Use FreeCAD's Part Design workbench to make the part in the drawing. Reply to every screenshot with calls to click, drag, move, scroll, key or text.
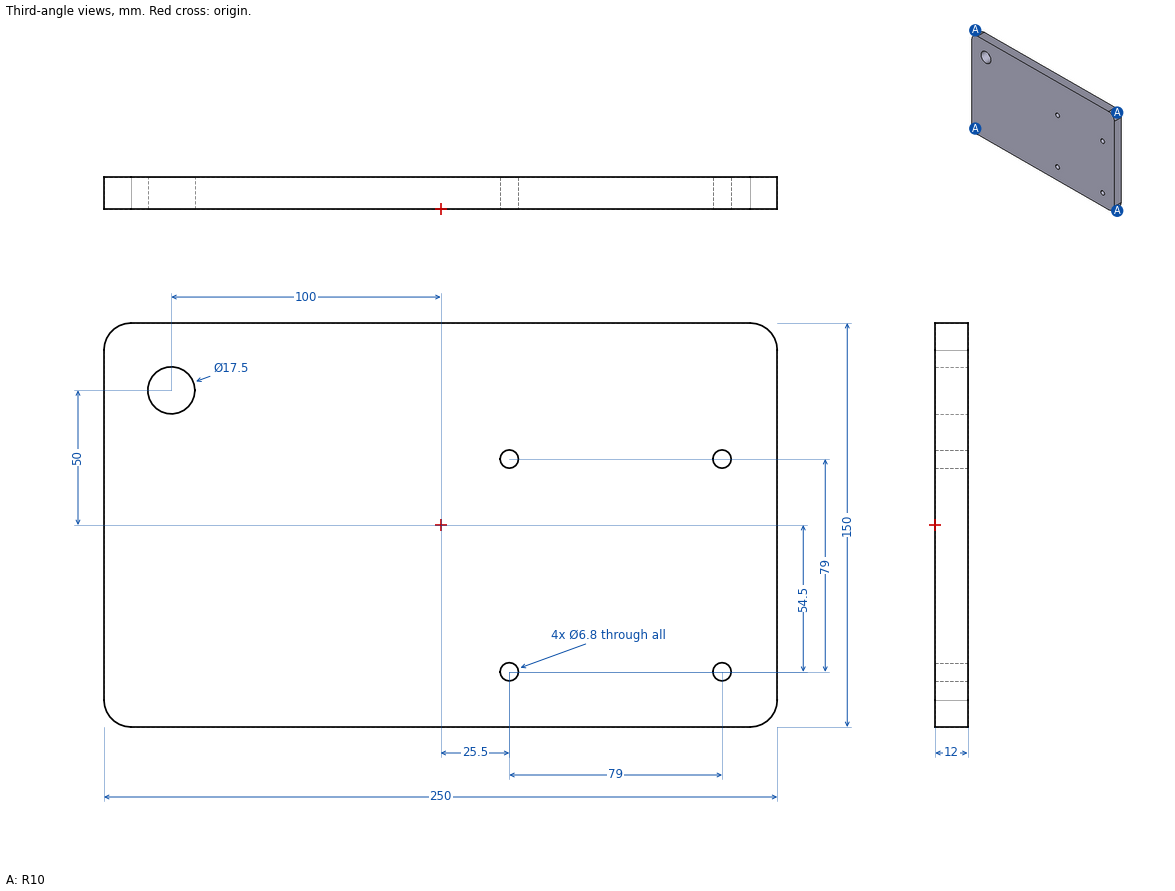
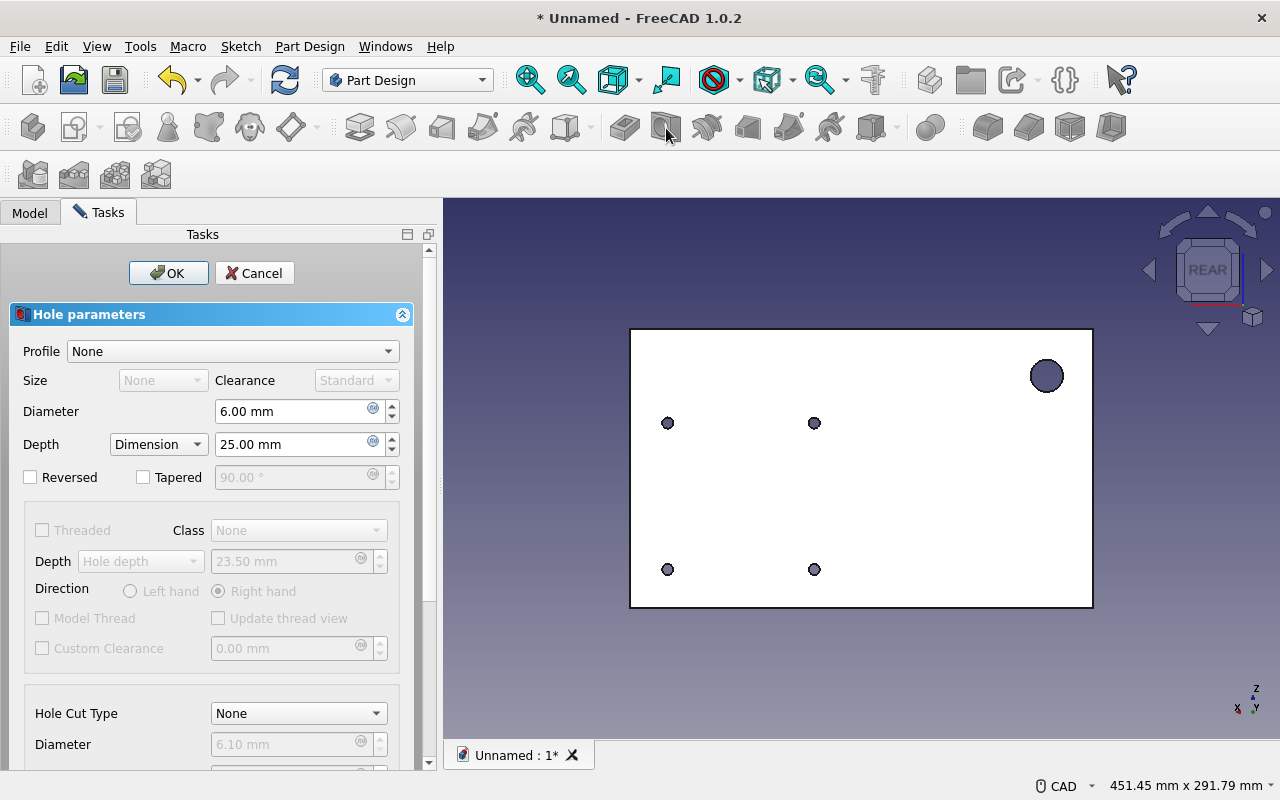
triple_click(300, 412)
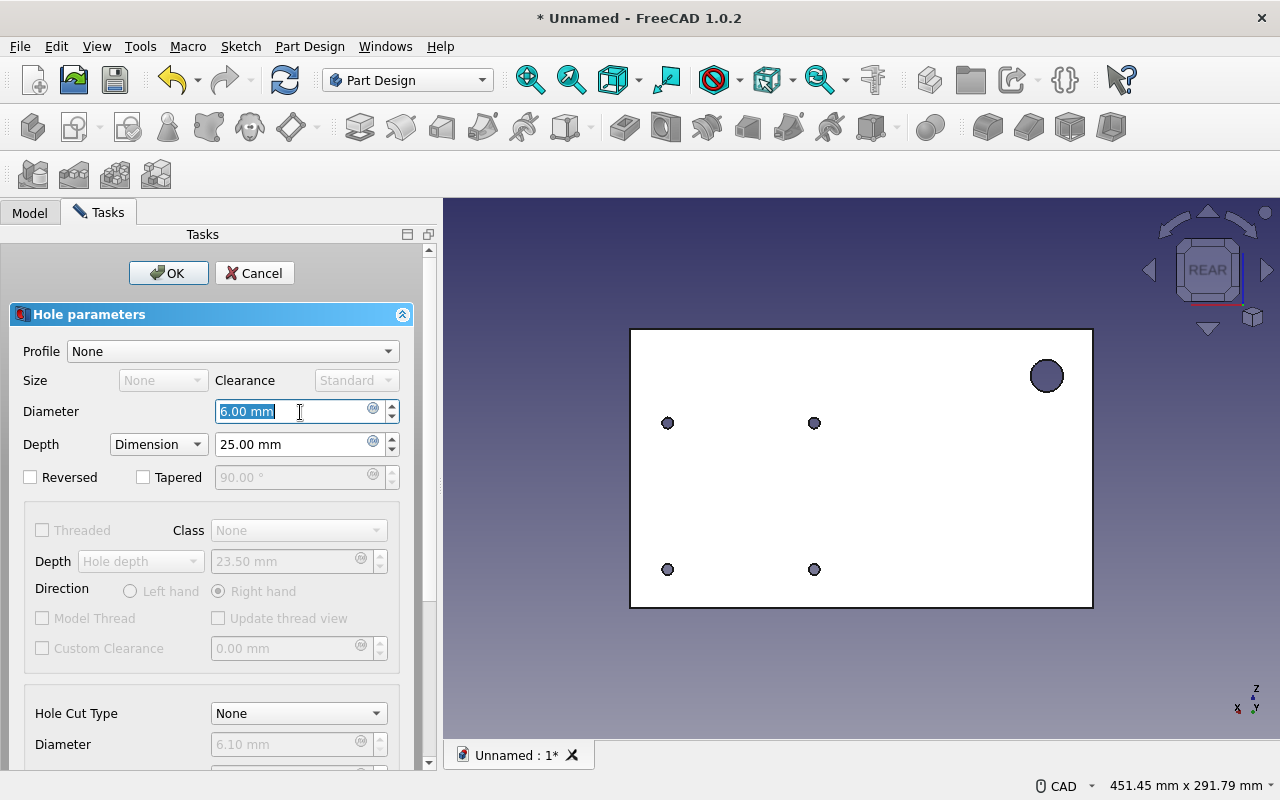
text(6.8)
key(Tab)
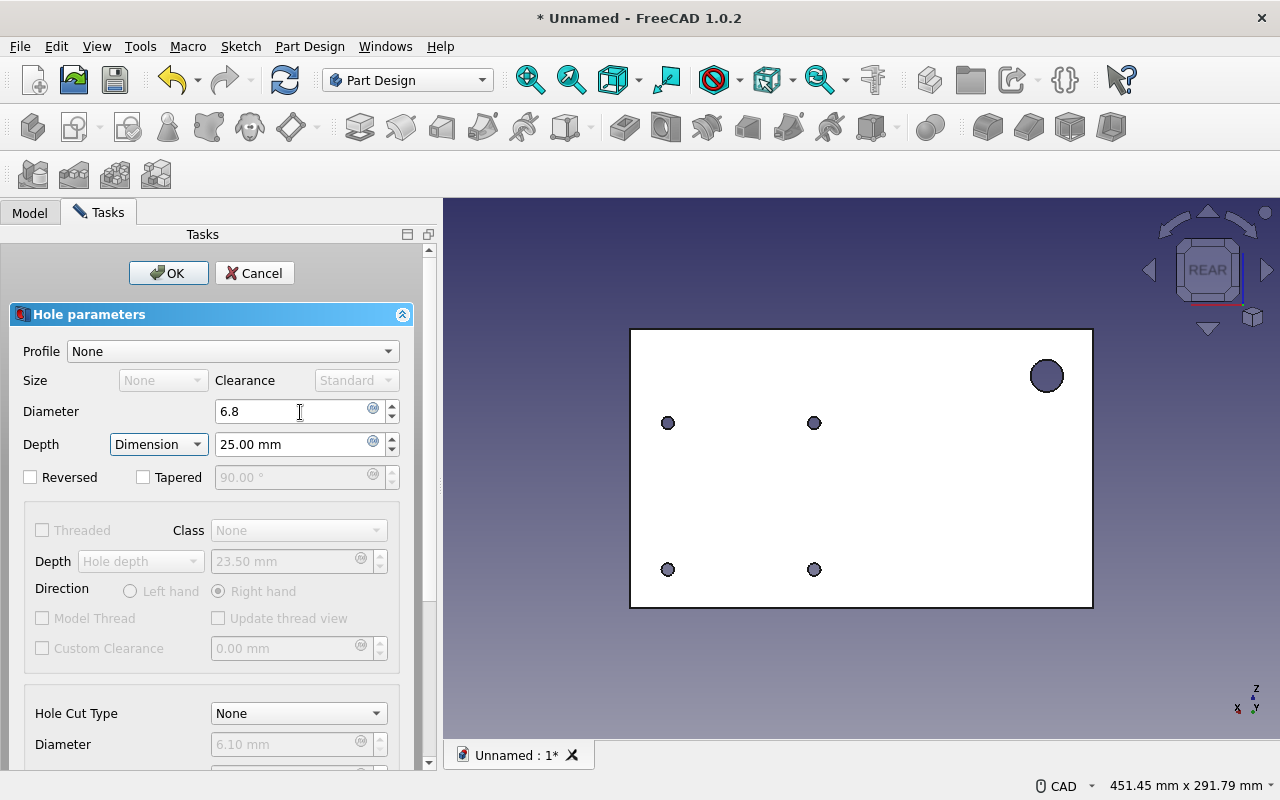
click(160, 444)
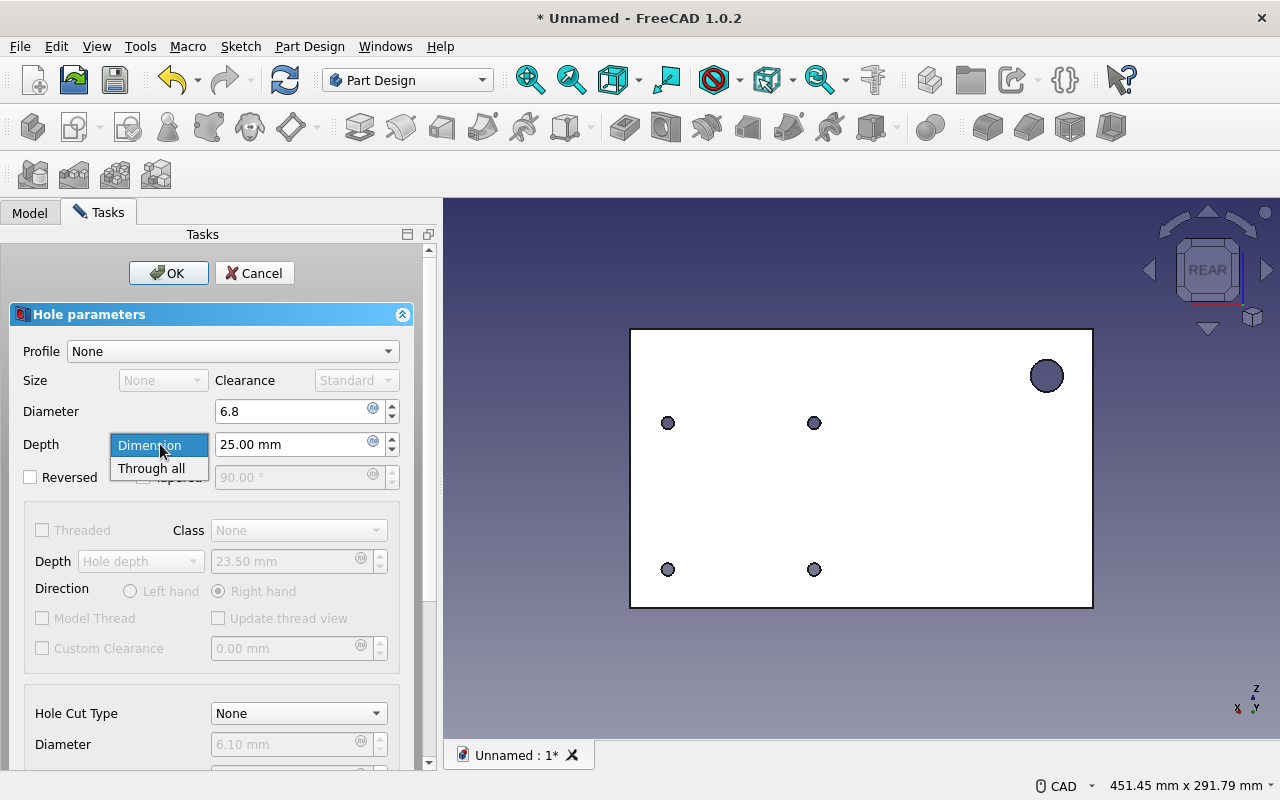
click(158, 468)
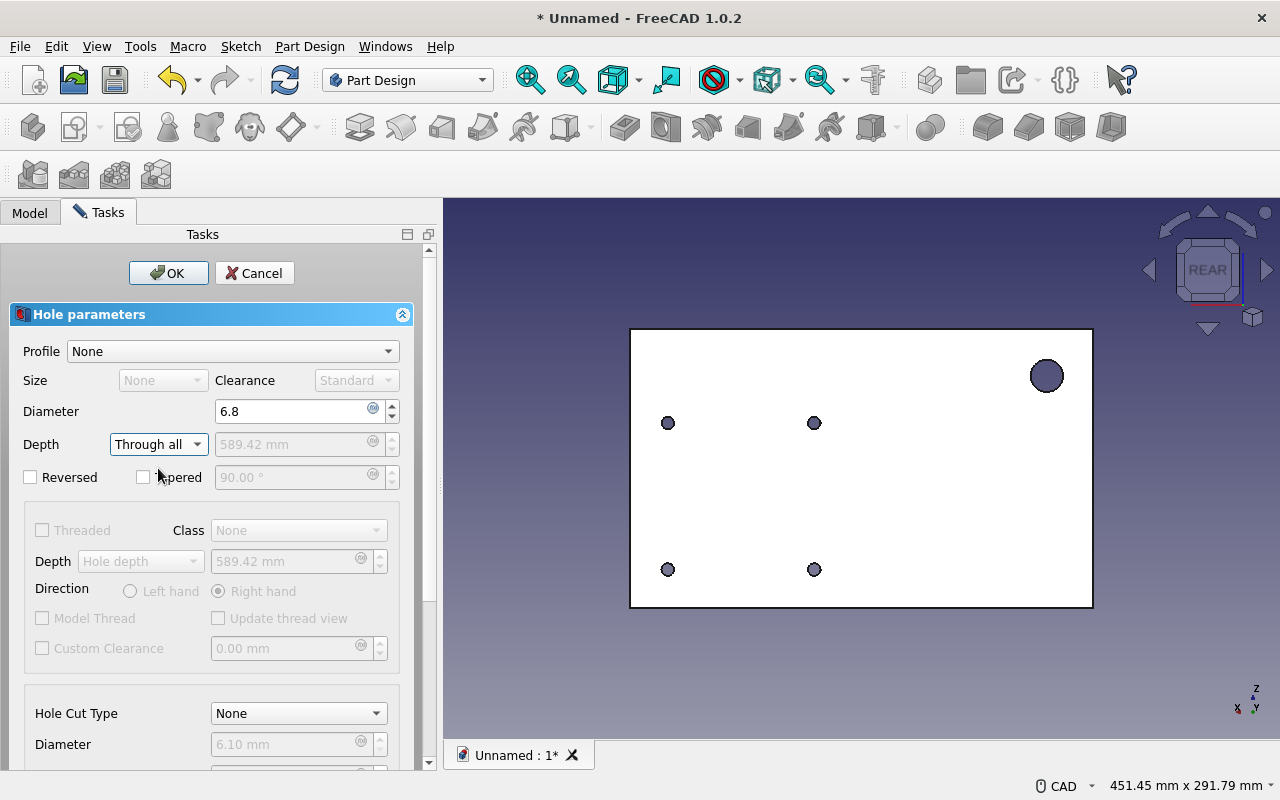
click(169, 273)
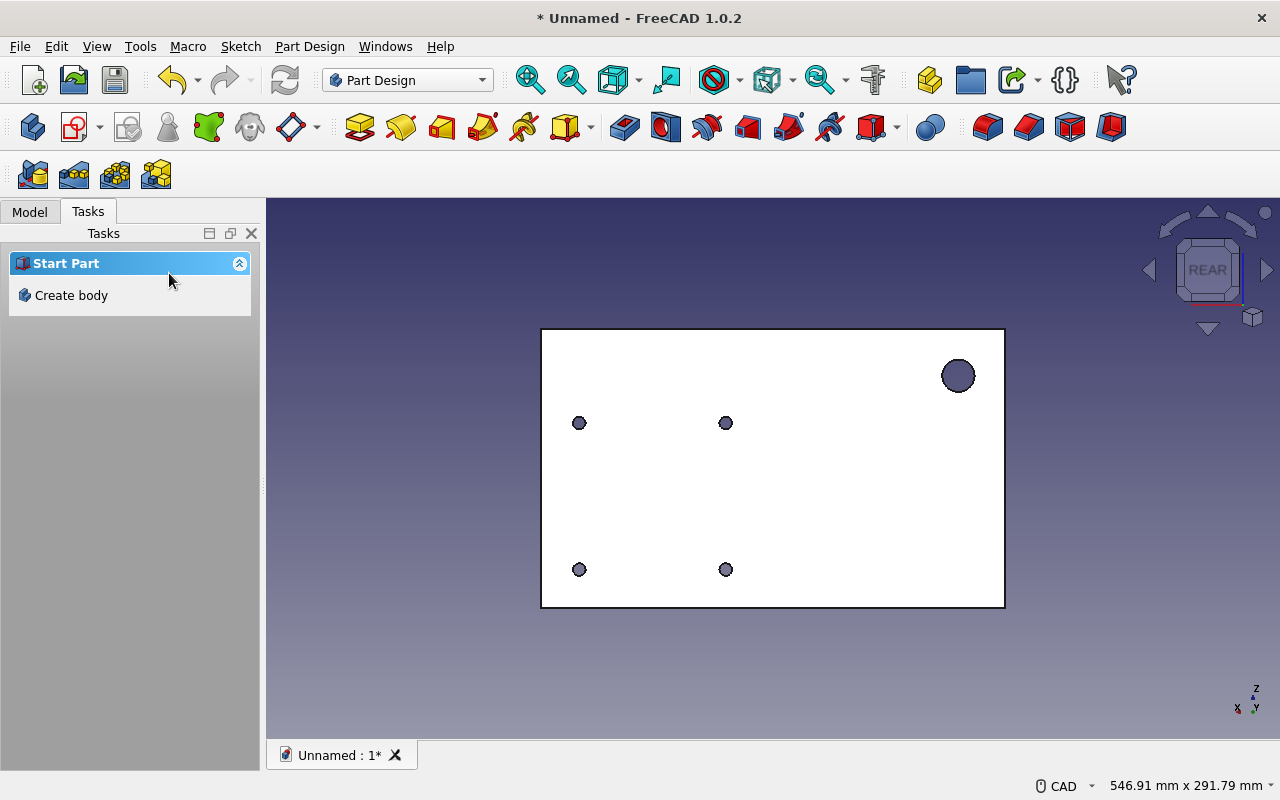
key(0)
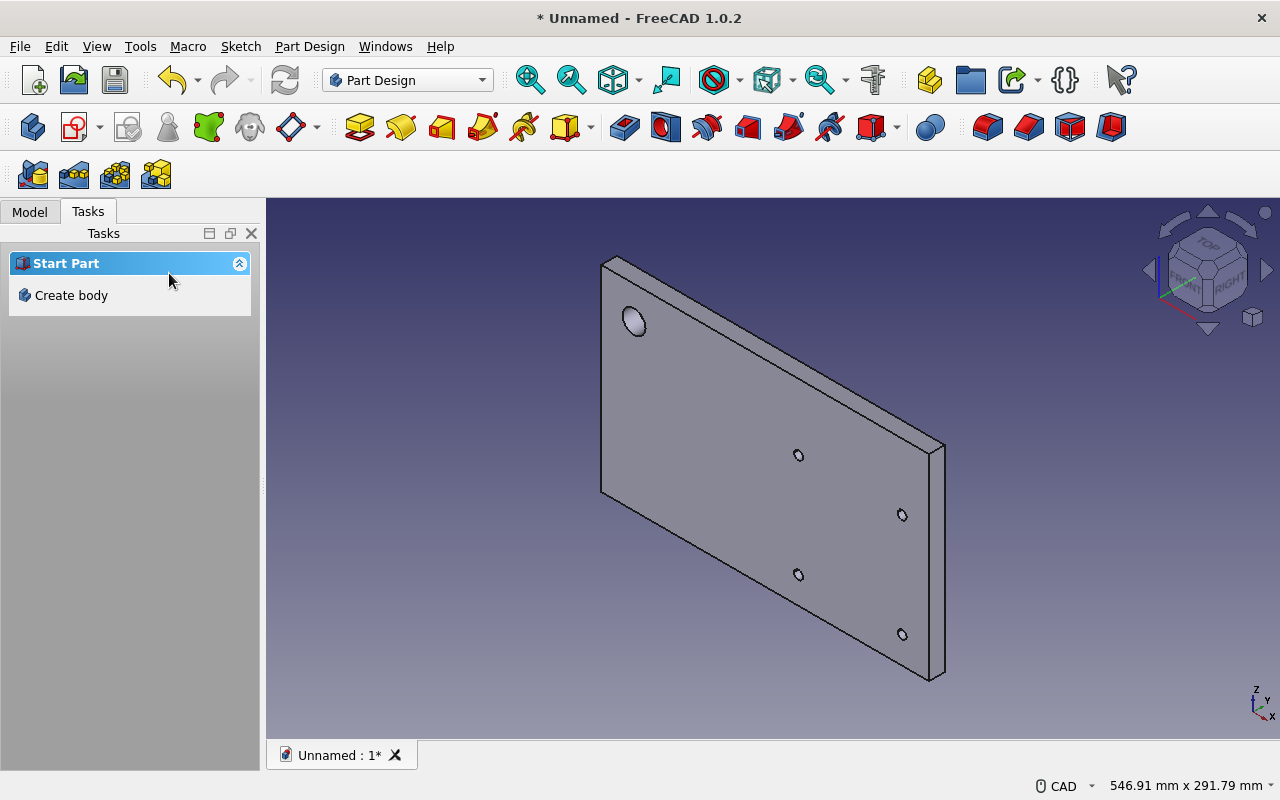
click(937, 449)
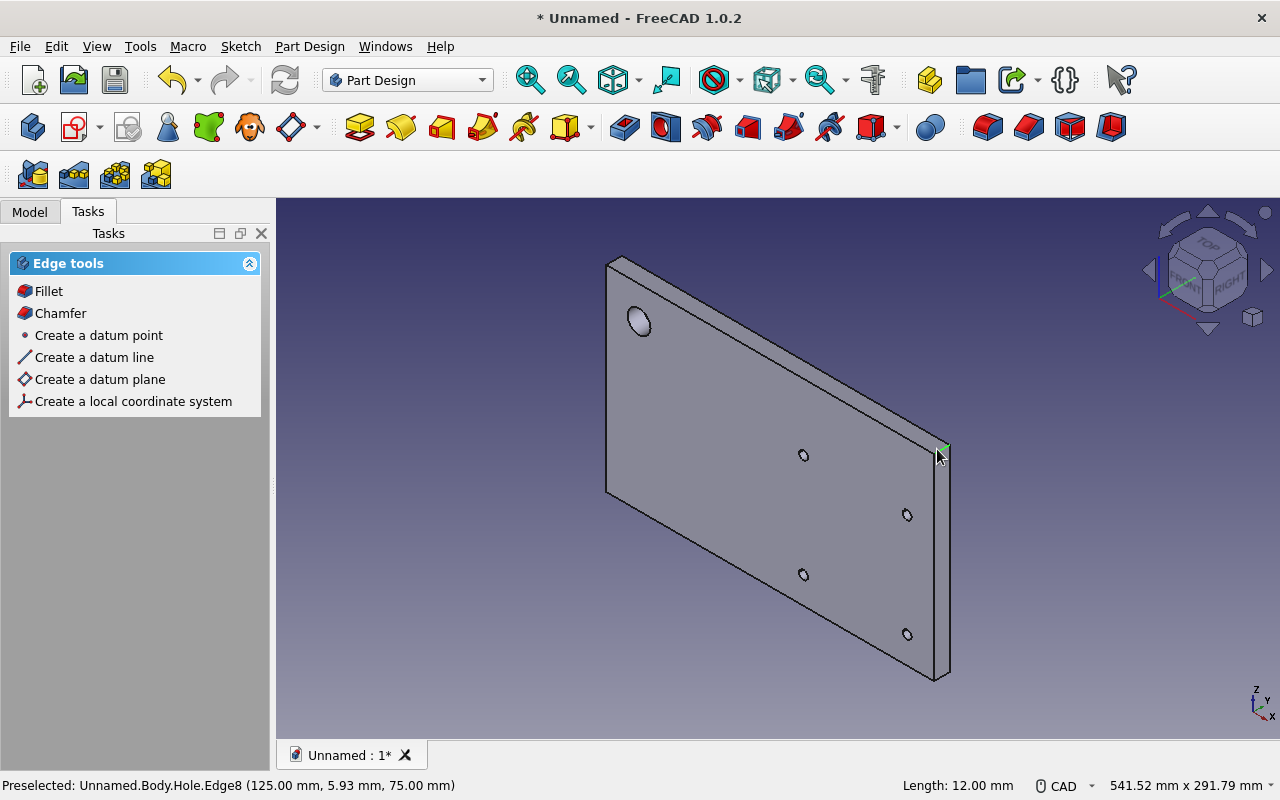
key(2)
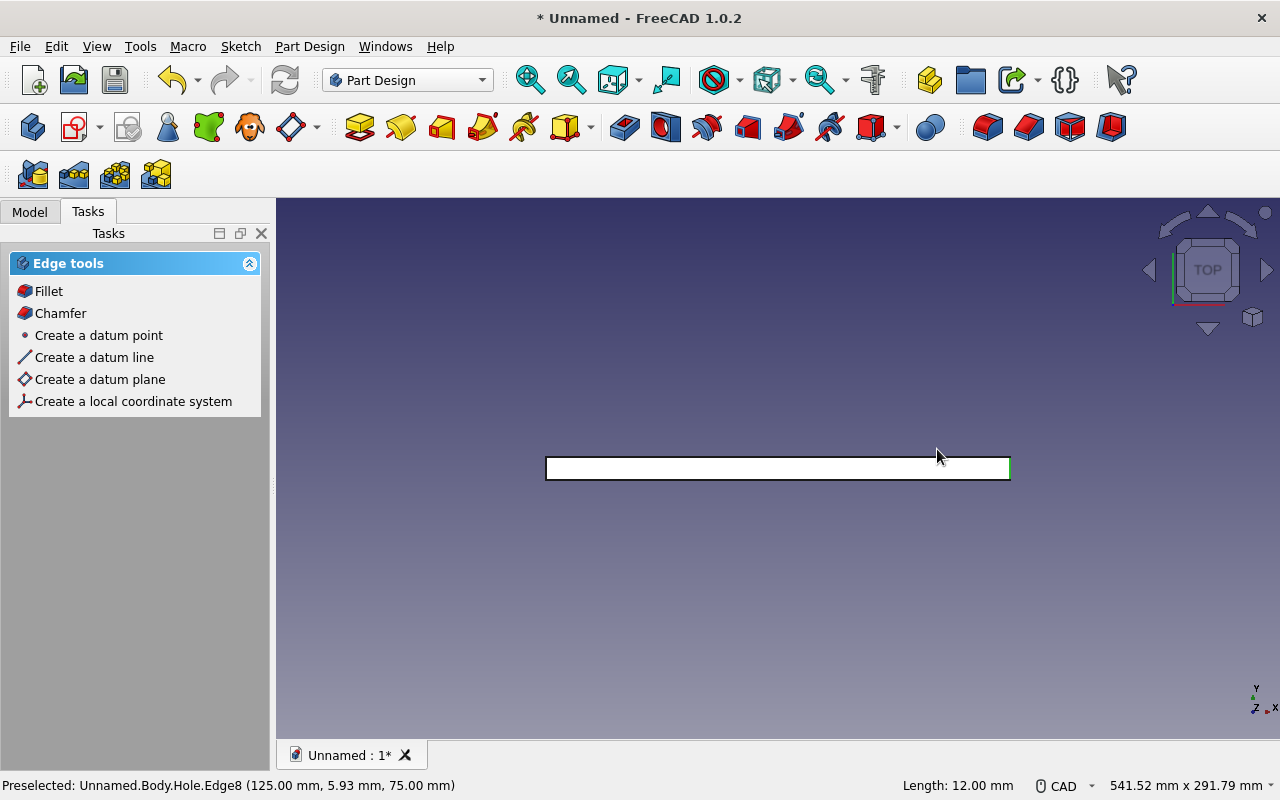
click(546, 467, ctrl)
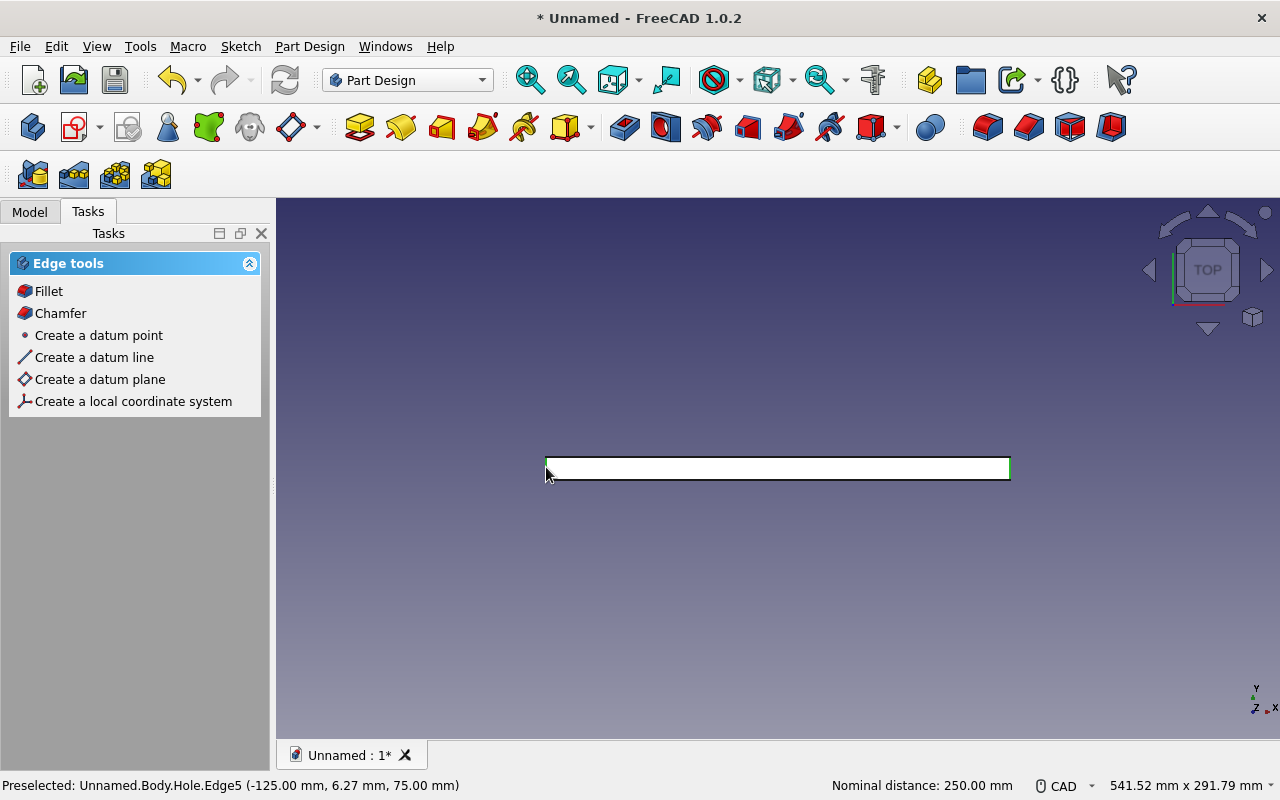
key(1)